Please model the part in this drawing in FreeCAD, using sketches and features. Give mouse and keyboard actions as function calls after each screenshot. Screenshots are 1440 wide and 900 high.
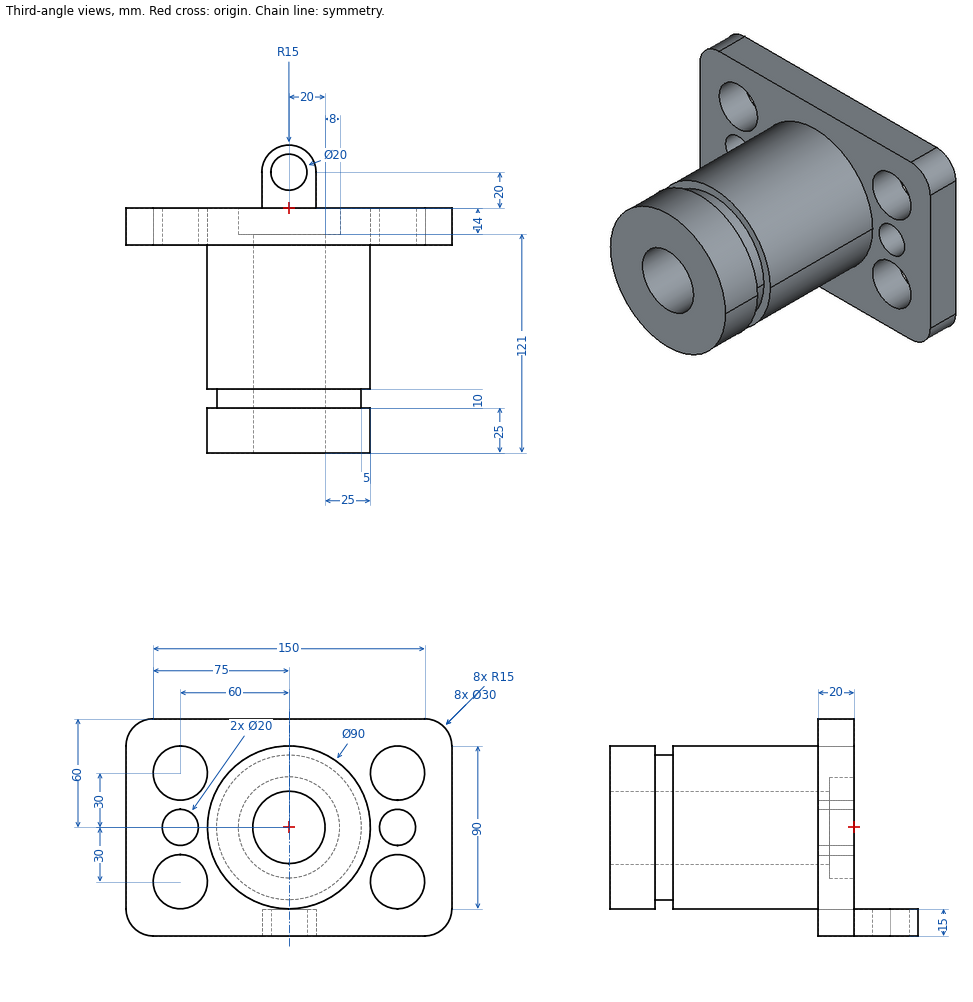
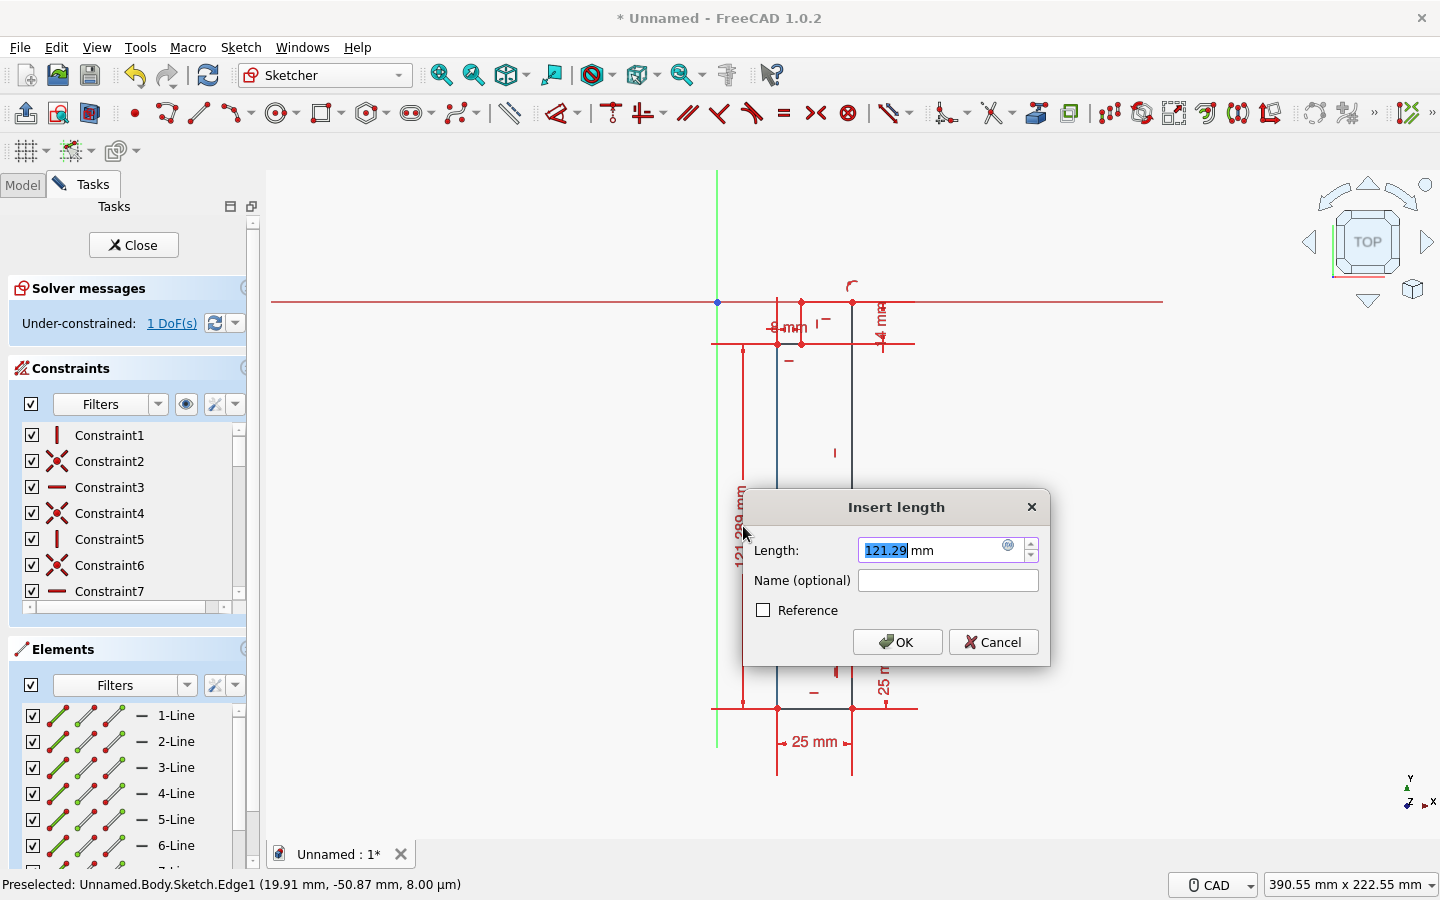
text(121)
key(Return)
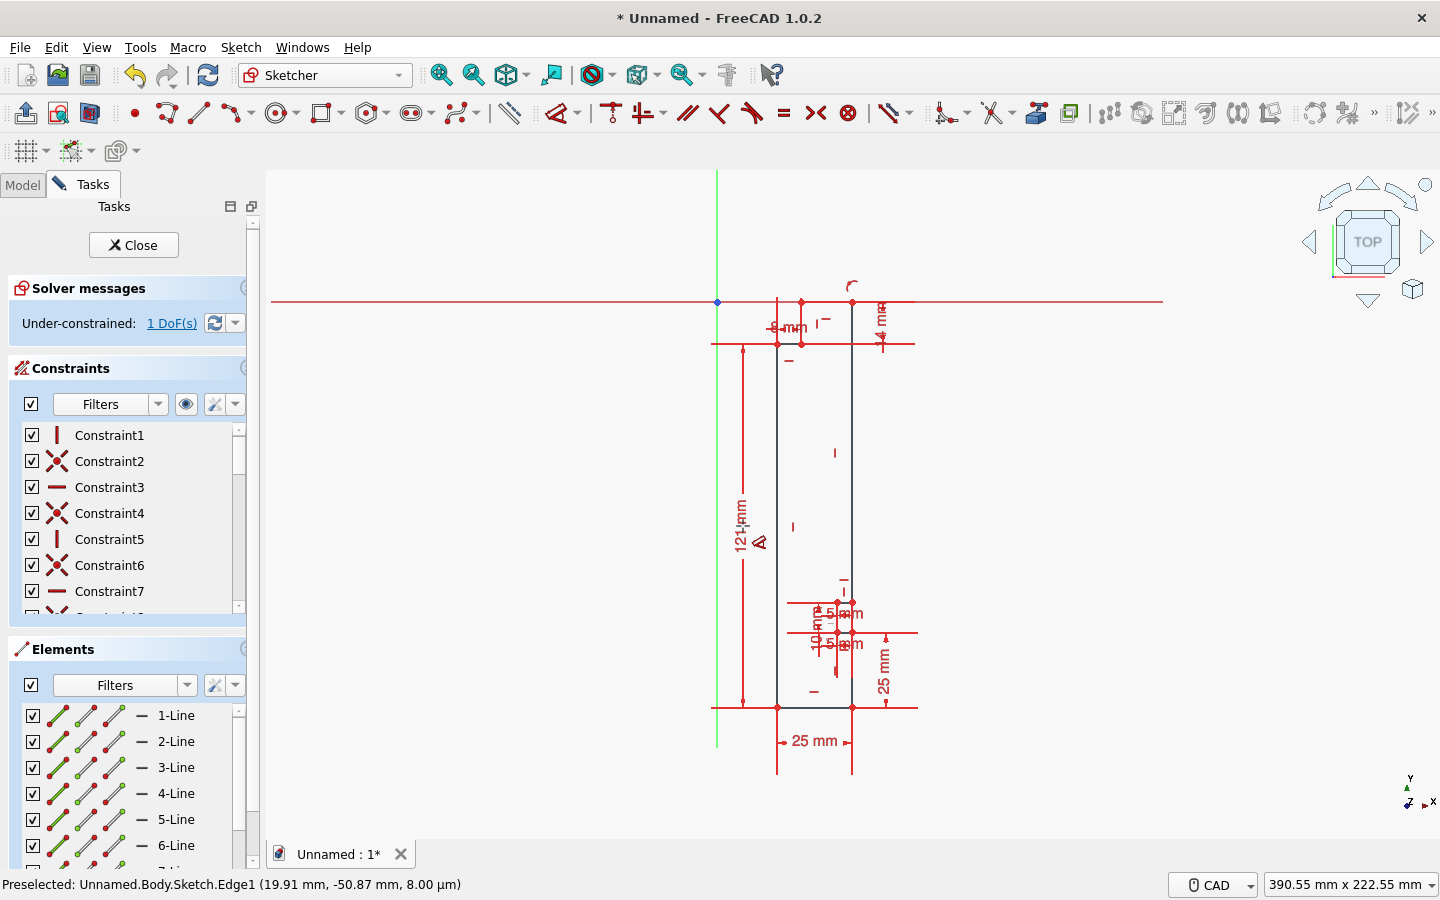
click(777, 344)
click(747, 268)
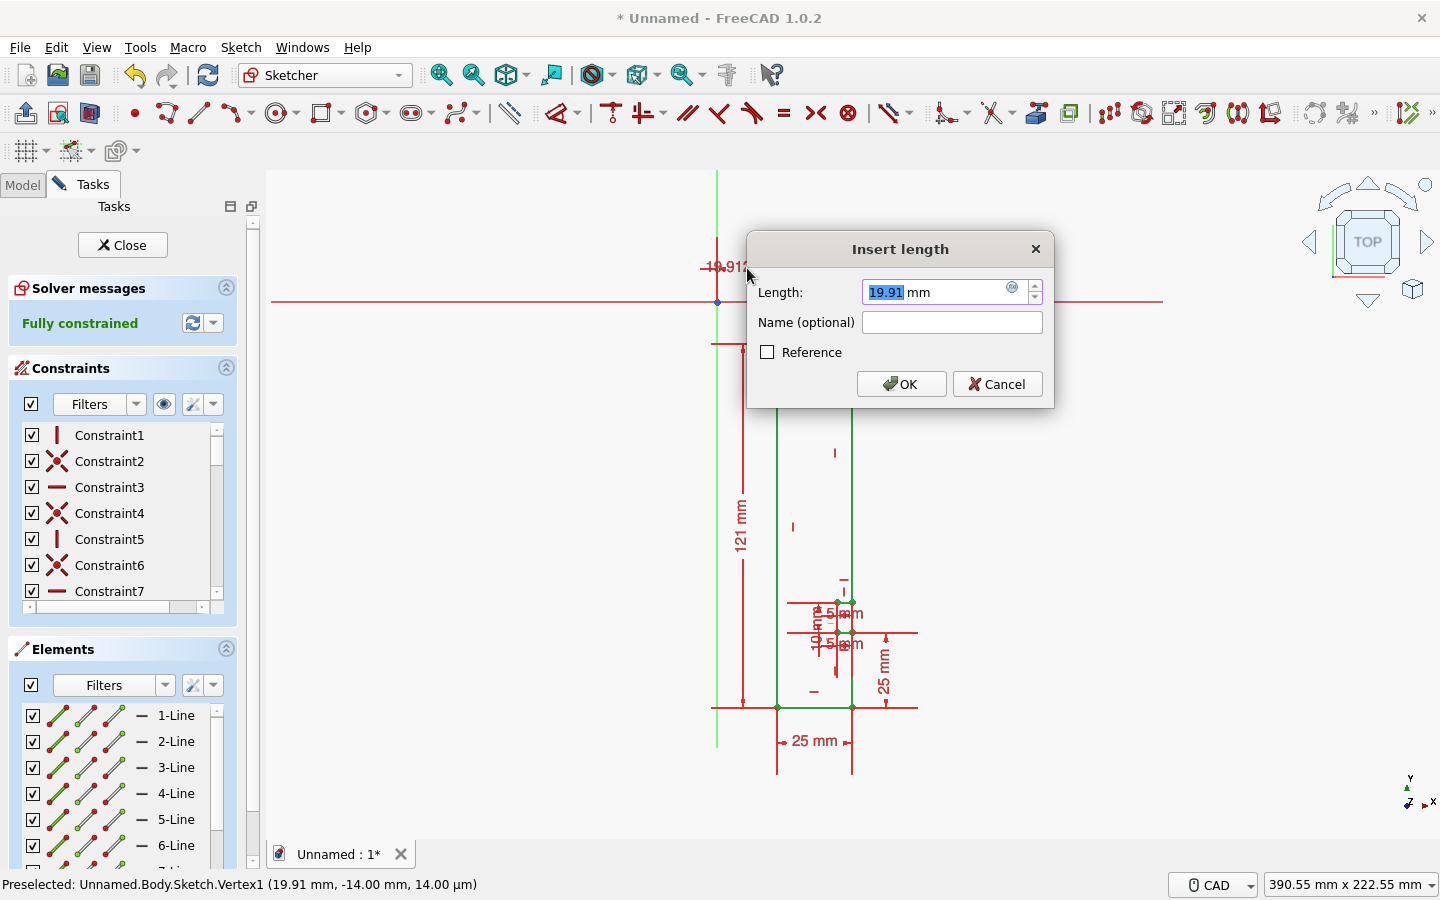
text(20)
key(Return)
key(Escape)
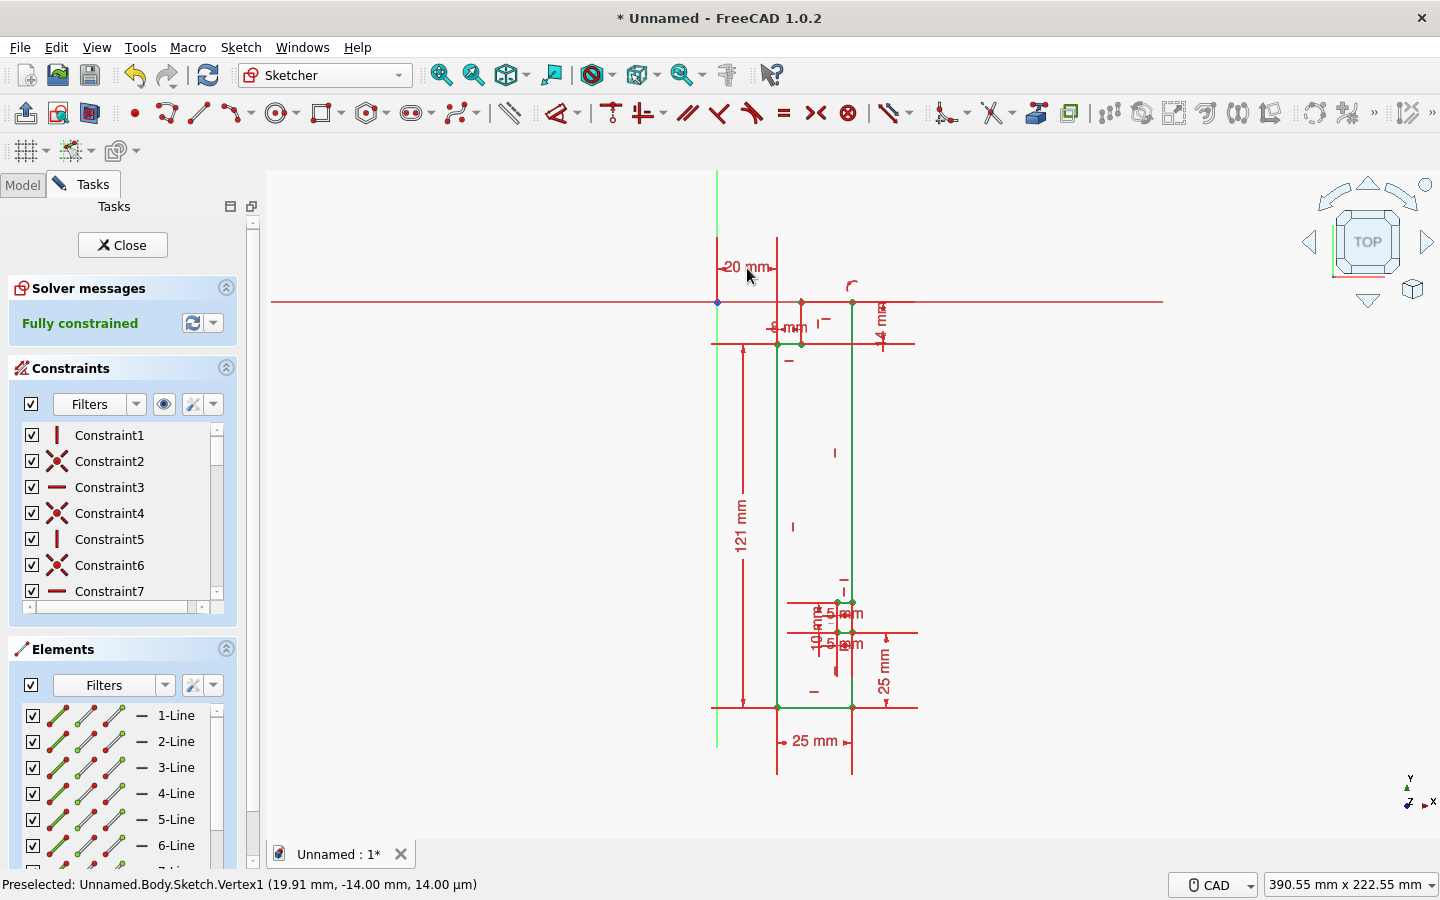
click(123, 245)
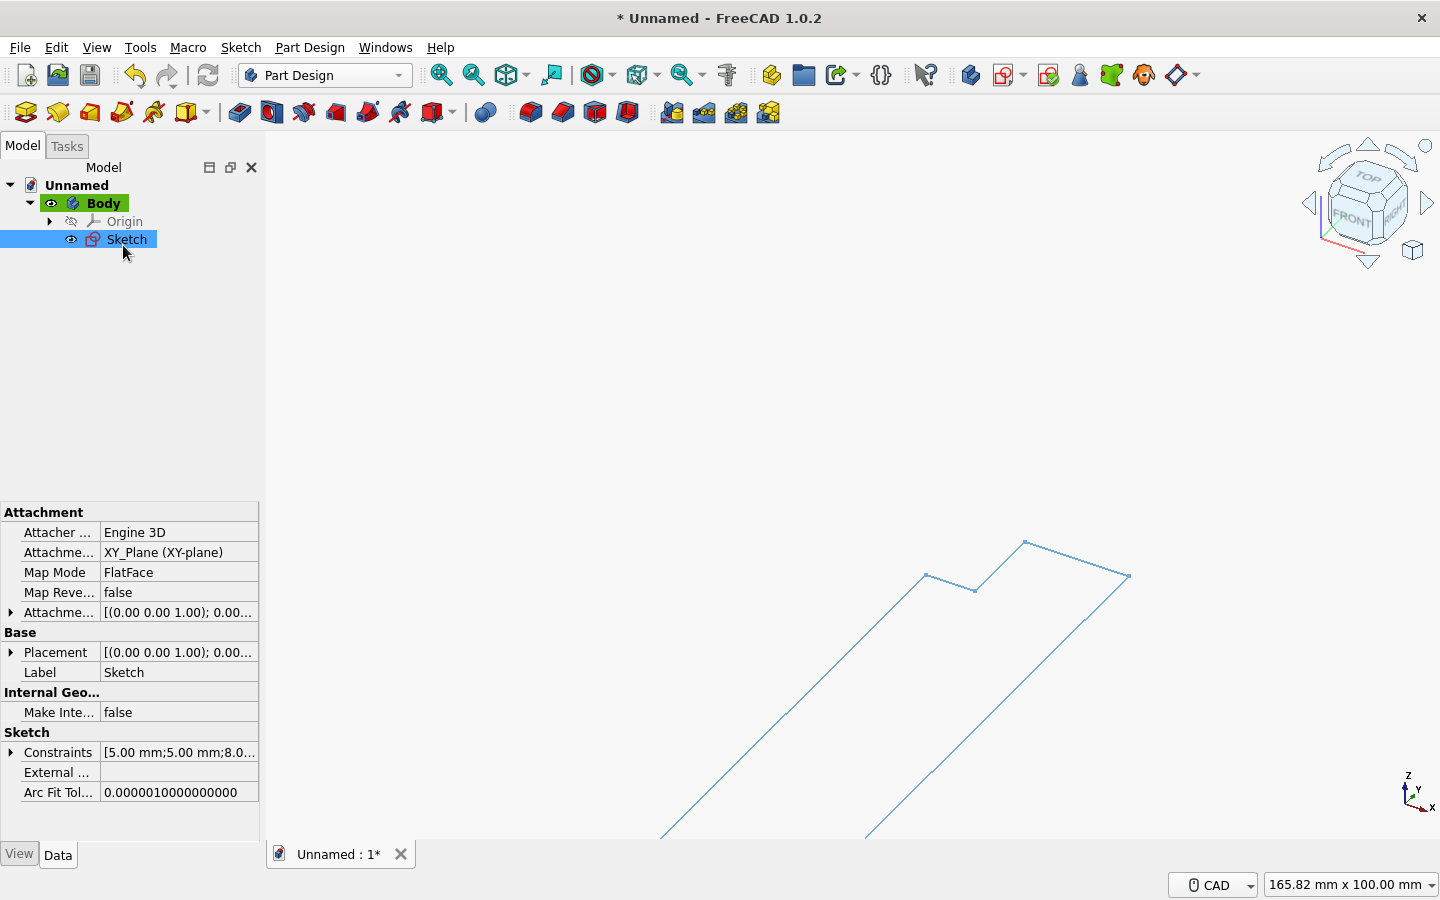
click(58, 112)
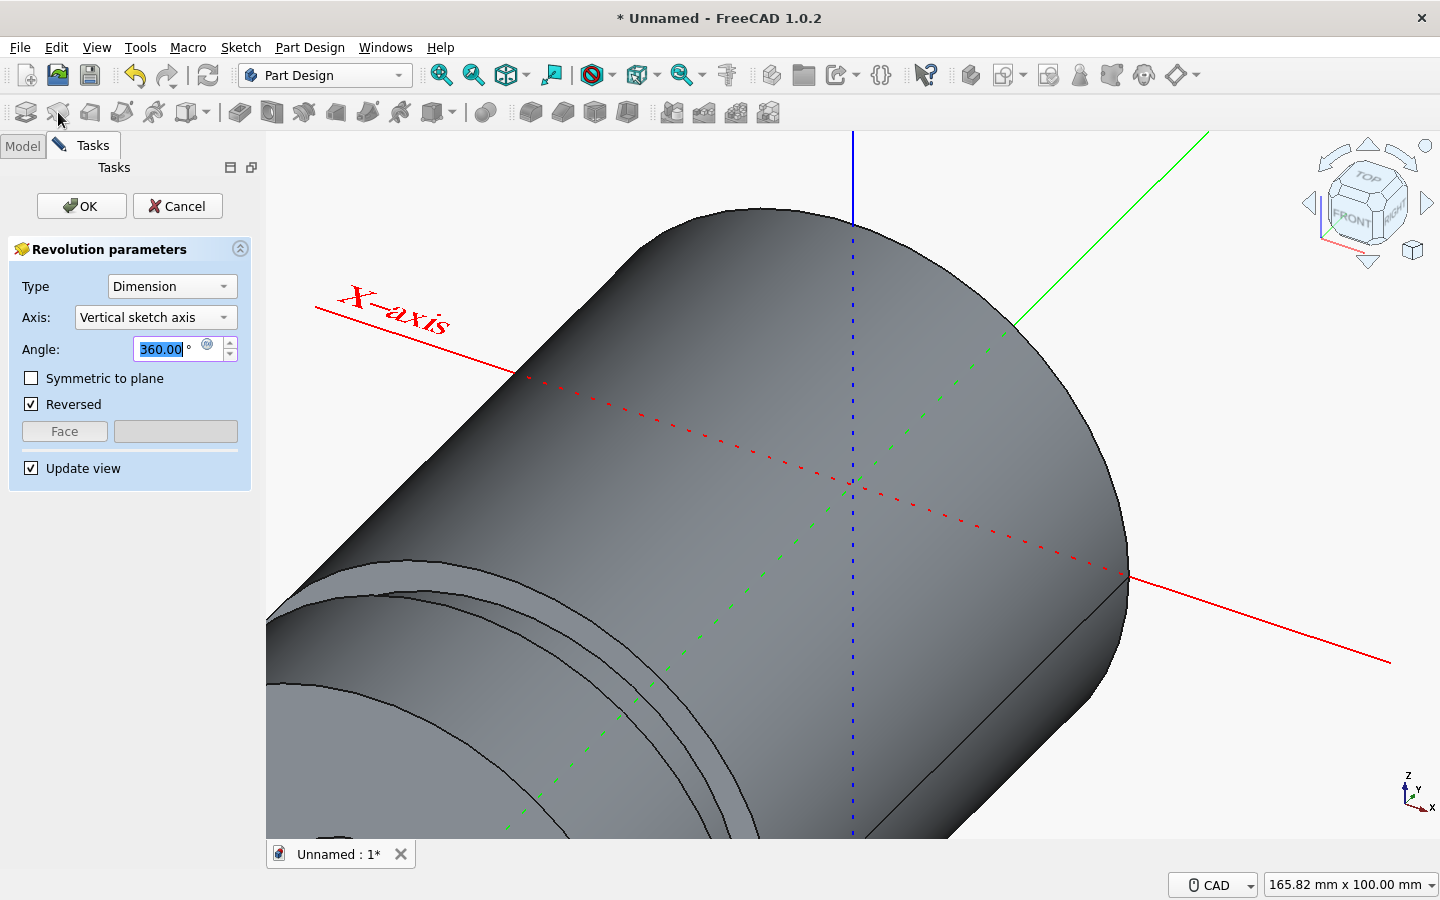
click(82, 206)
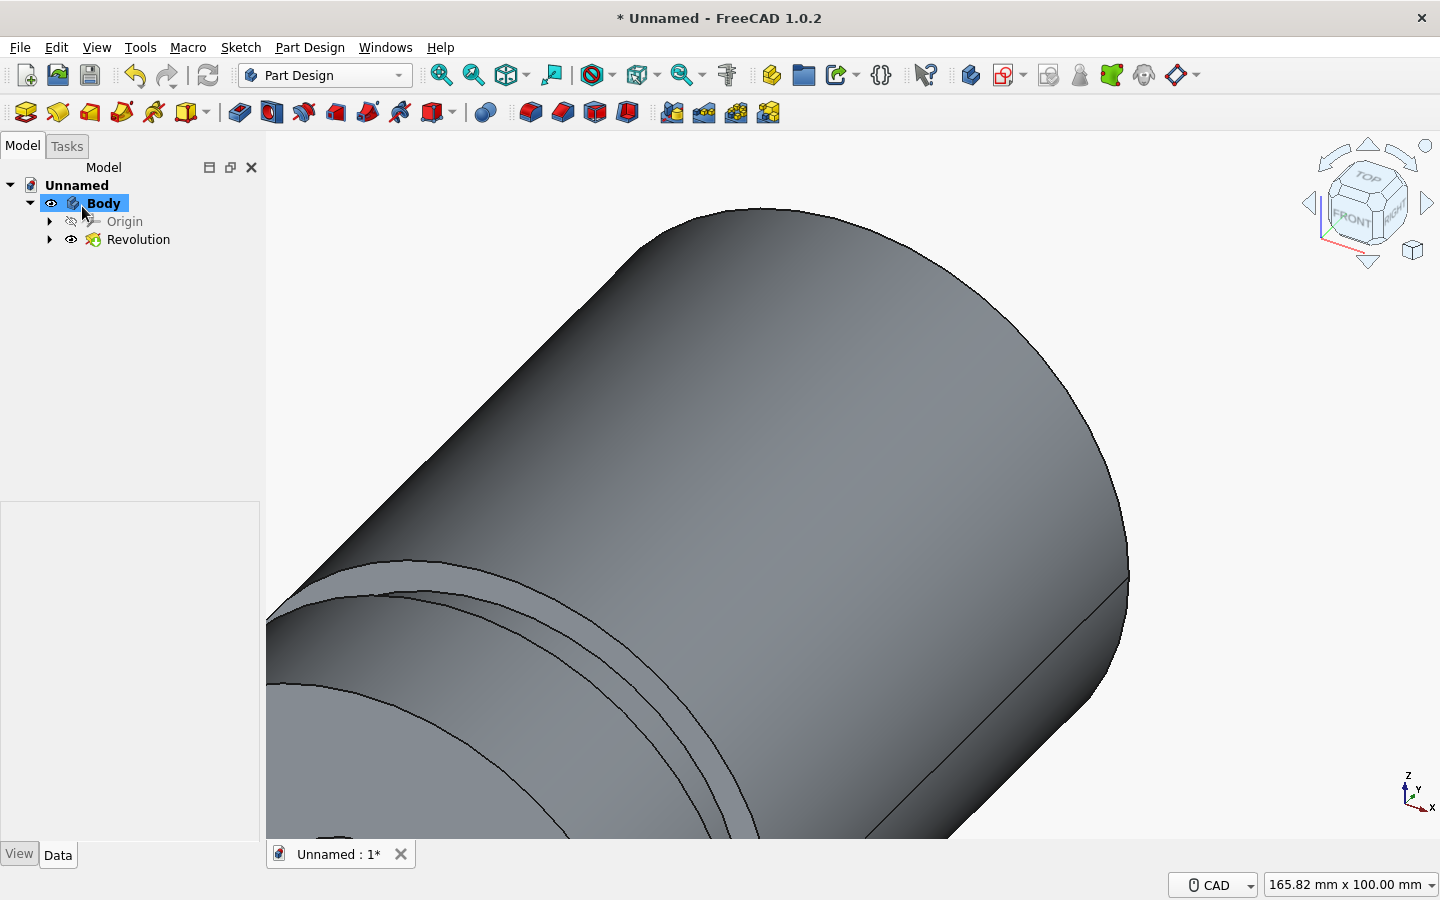
click(442, 76)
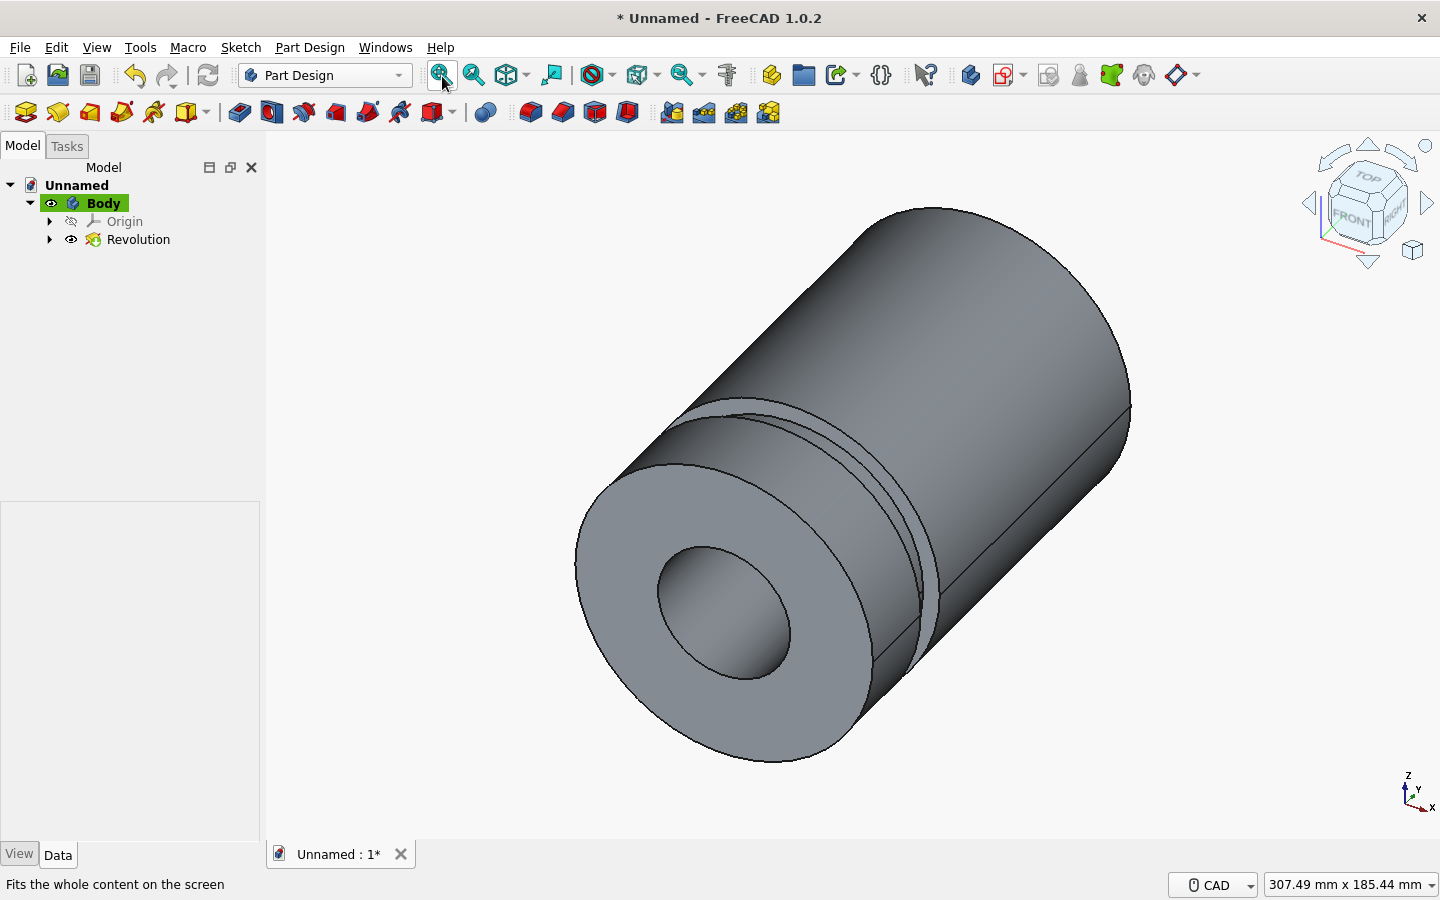
click(50, 221)